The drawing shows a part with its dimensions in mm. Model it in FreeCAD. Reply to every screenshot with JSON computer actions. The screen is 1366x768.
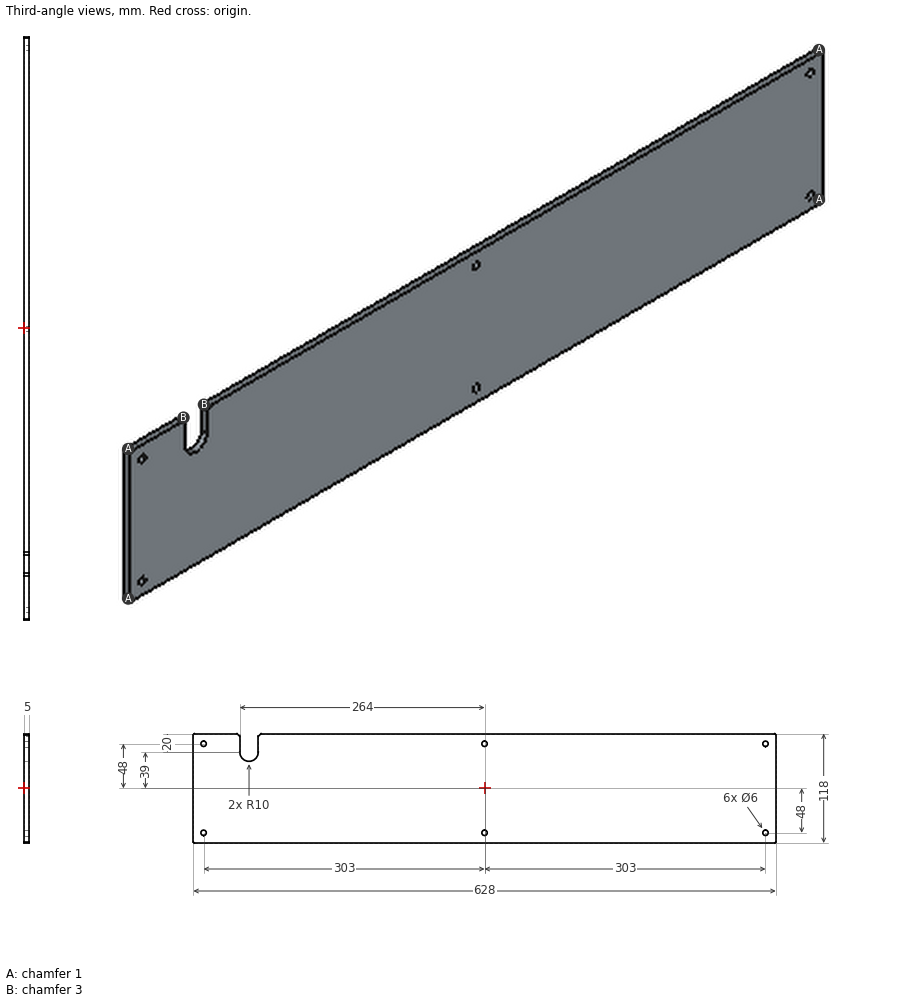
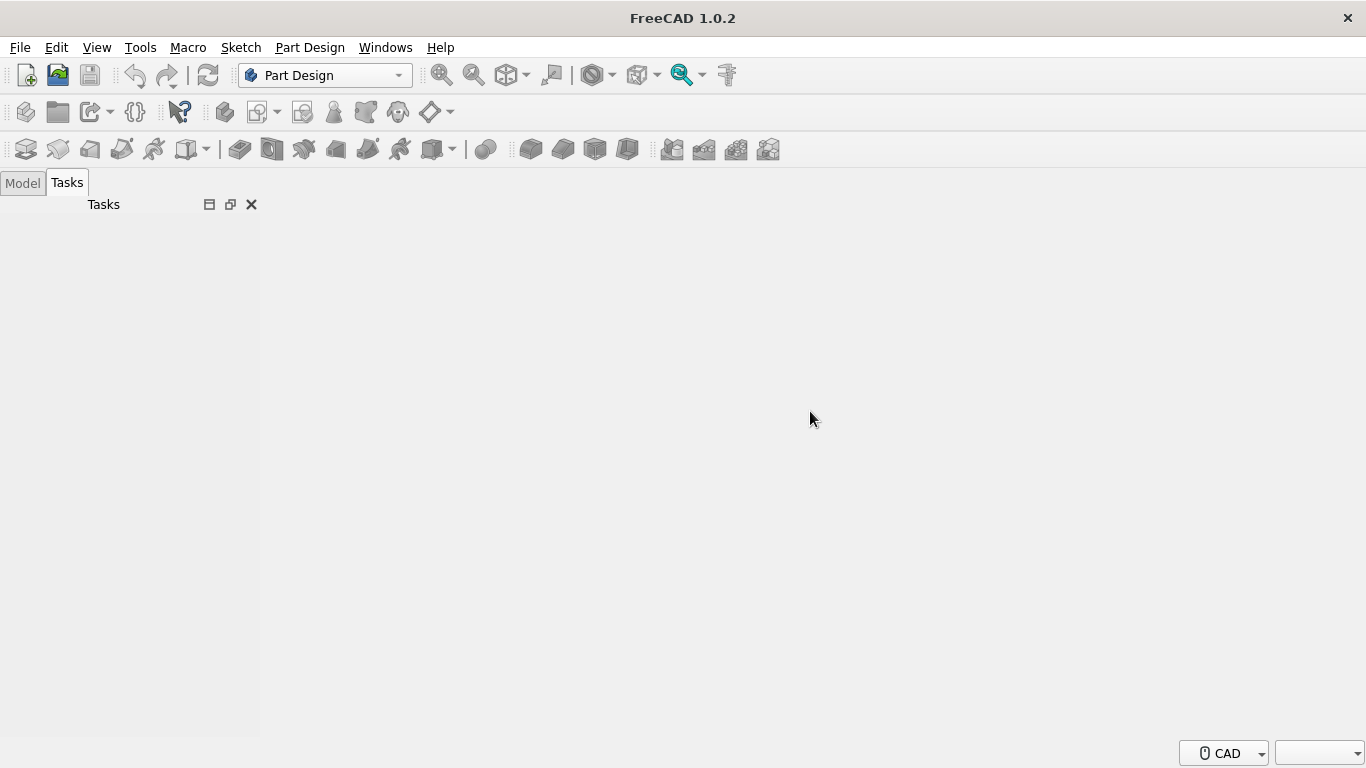
{"action": "key", "text": "ctrl+n"}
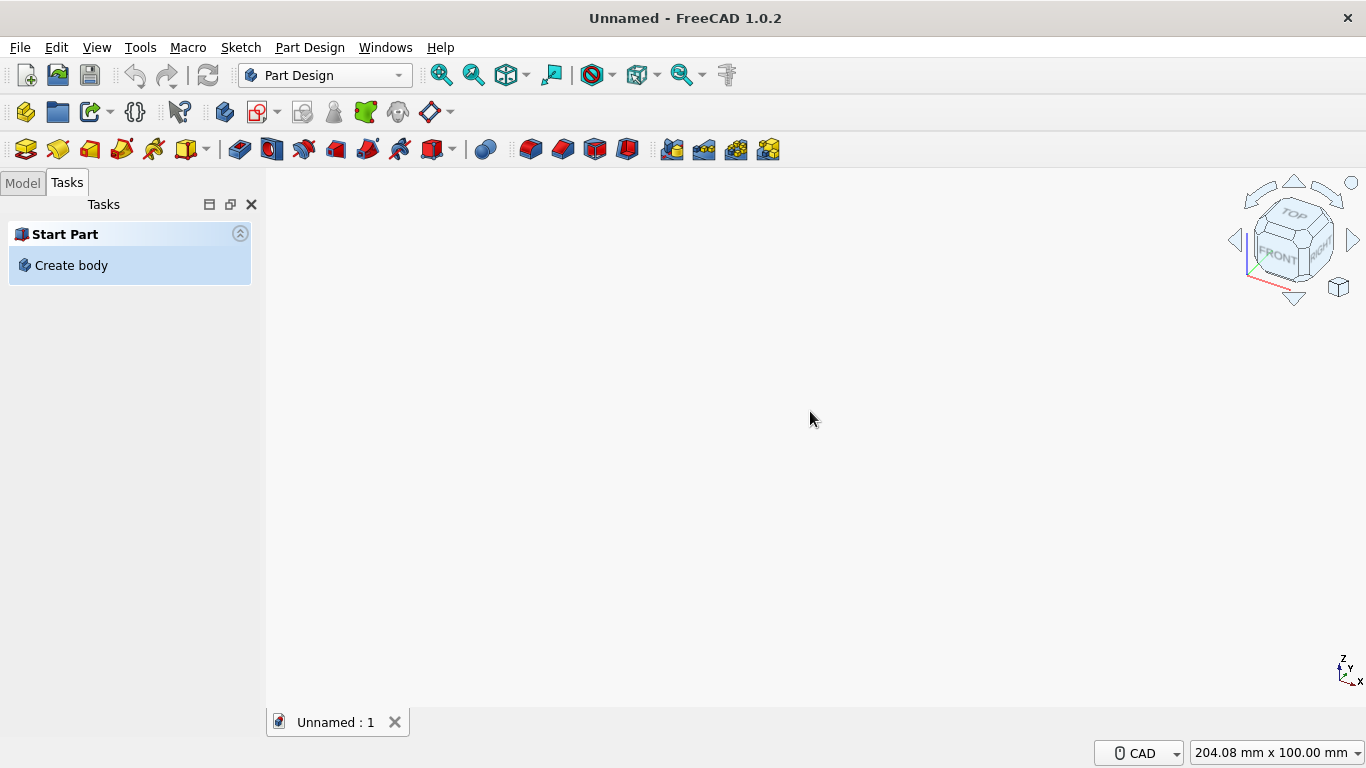
{"action": "left_click", "coordinate": [258, 112]}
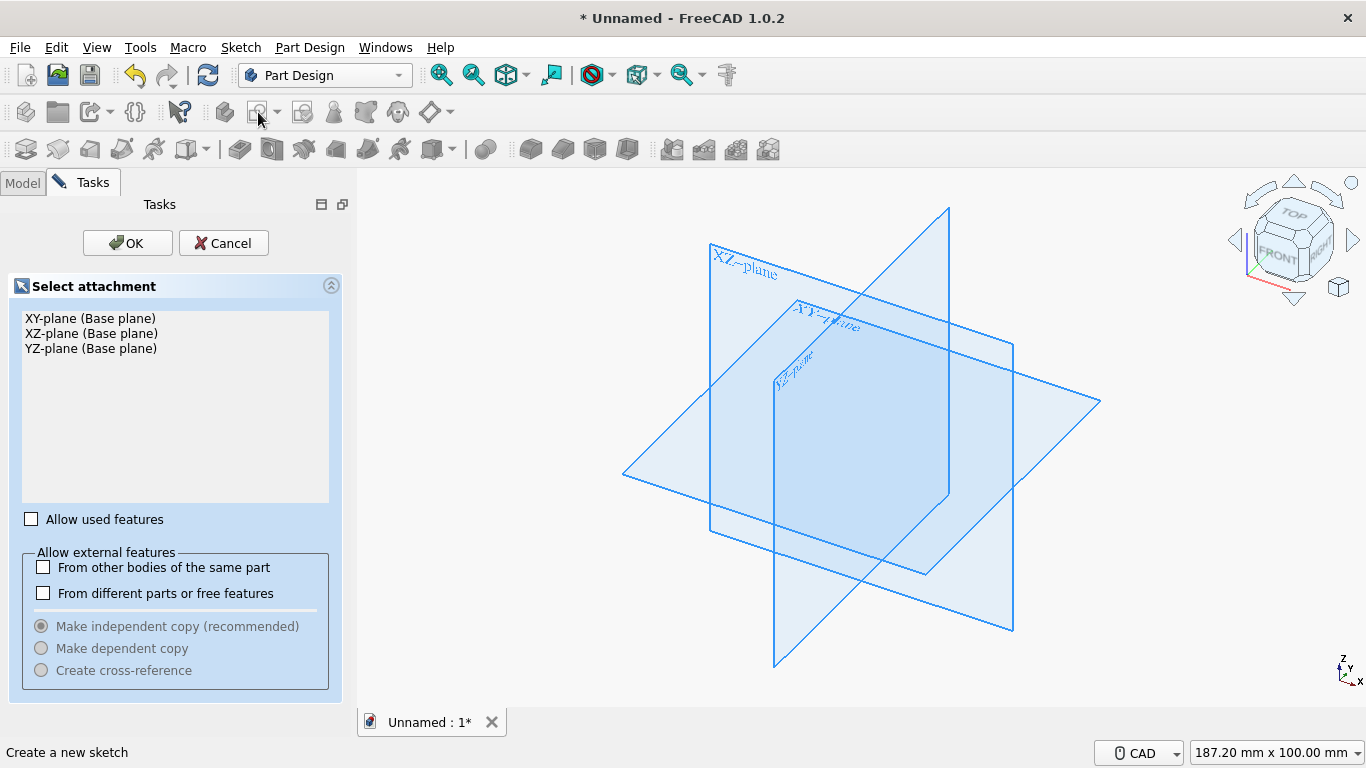
{"action": "left_click", "coordinate": [82, 348]}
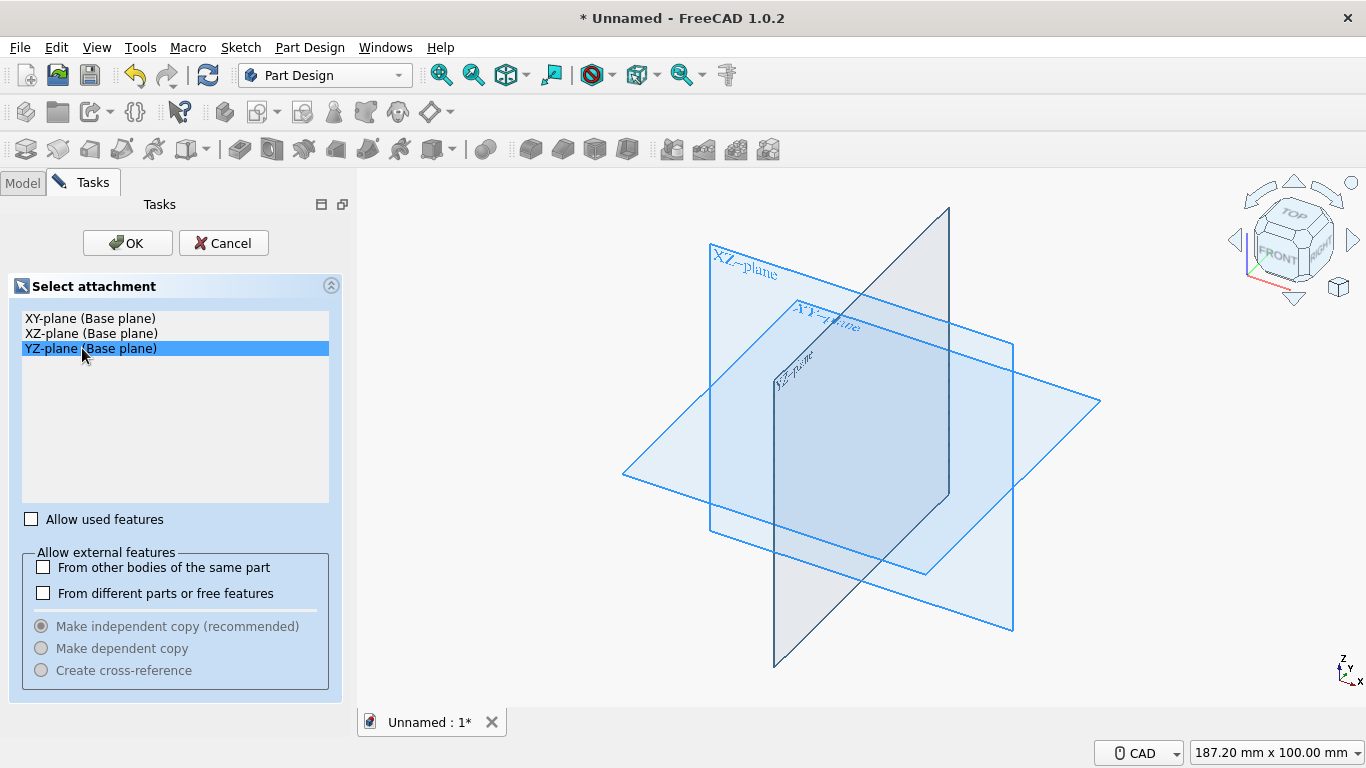
{"action": "left_click", "coordinate": [128, 243]}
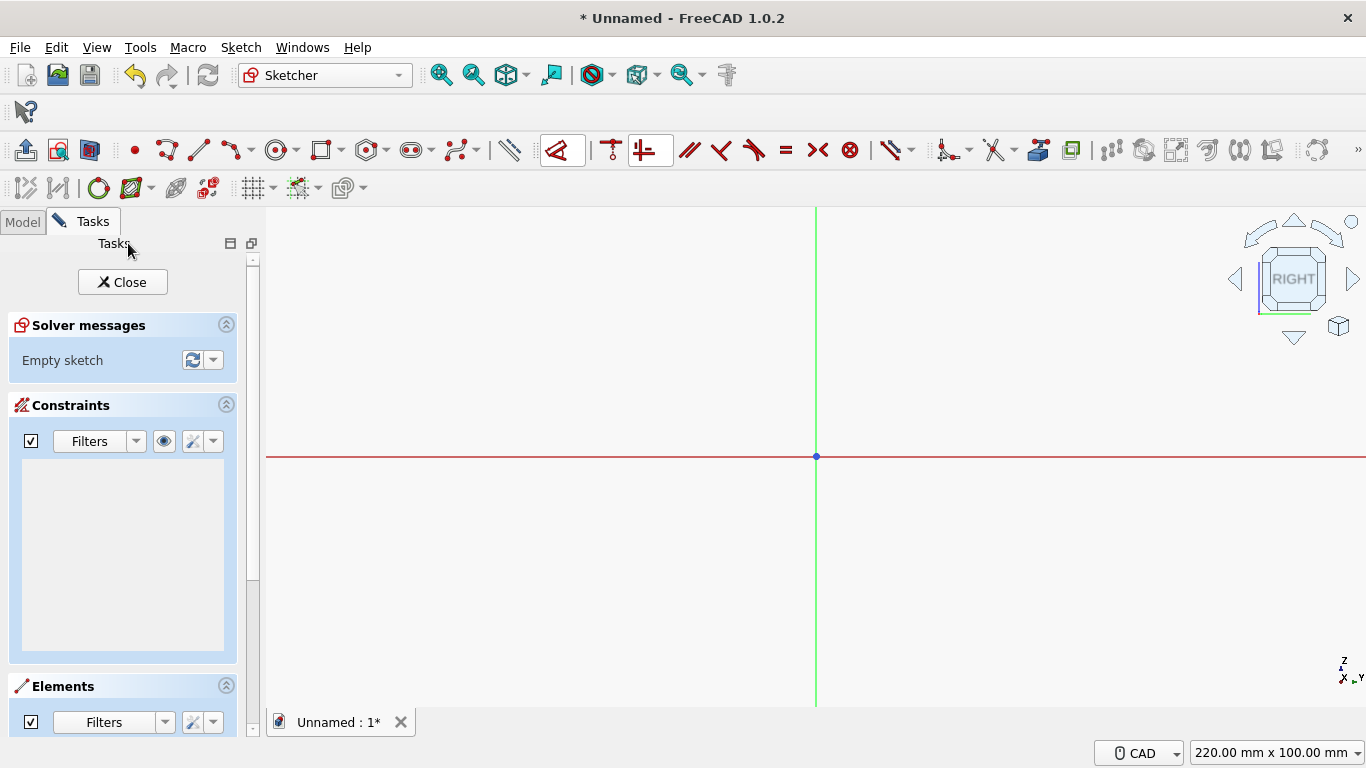
{"action": "scroll", "coordinate": [730, 457], "scroll_direction": "down", "scroll_amount": 8}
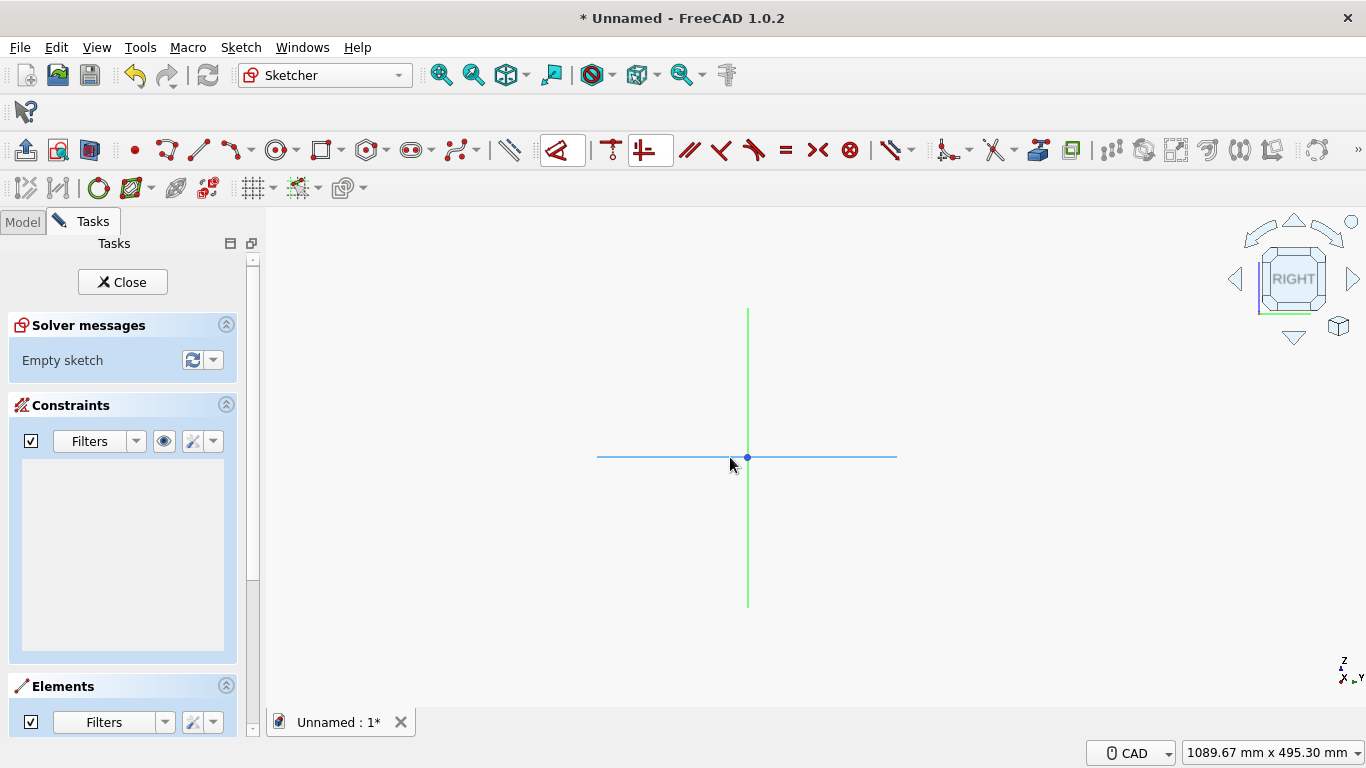
{"action": "key", "text": "g v"}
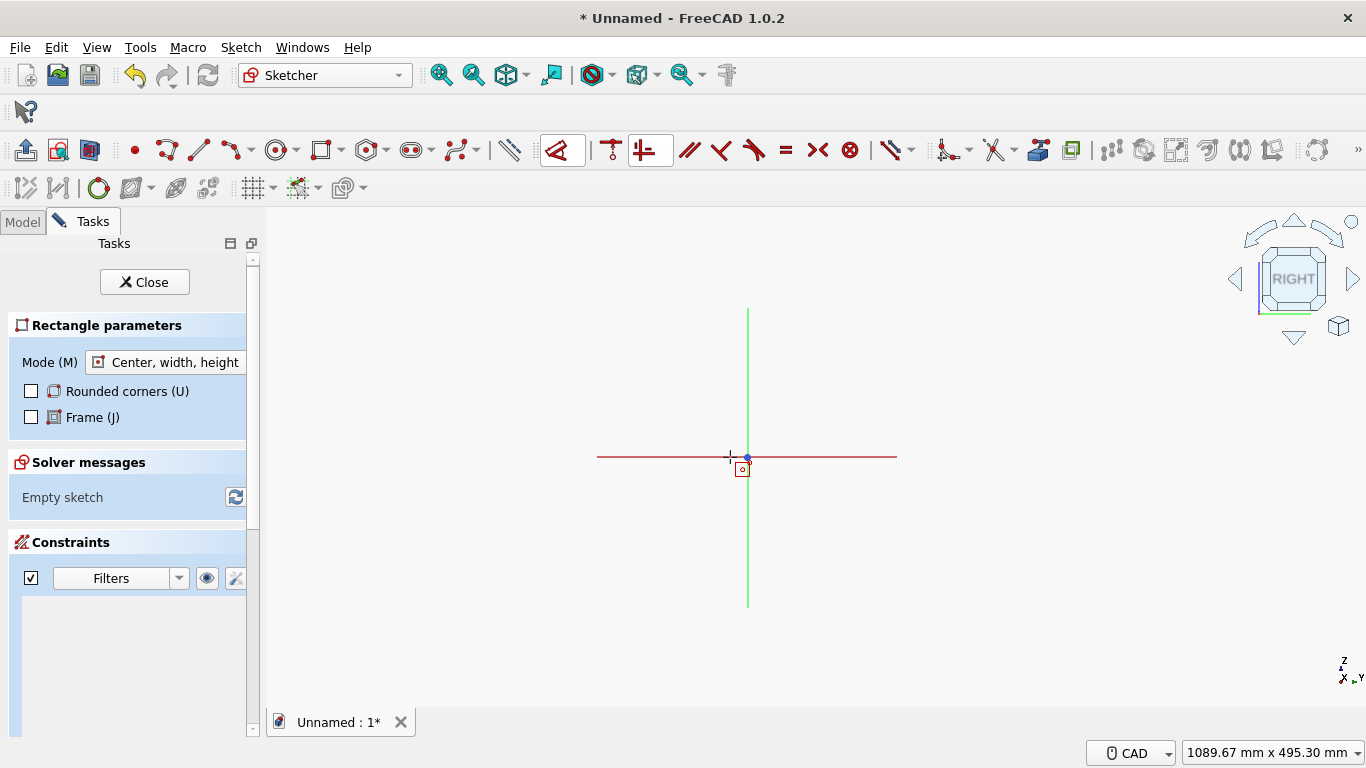
{"action": "left_click", "coordinate": [748, 457]}
{"action": "mouse_move", "coordinate": [1065, 398]}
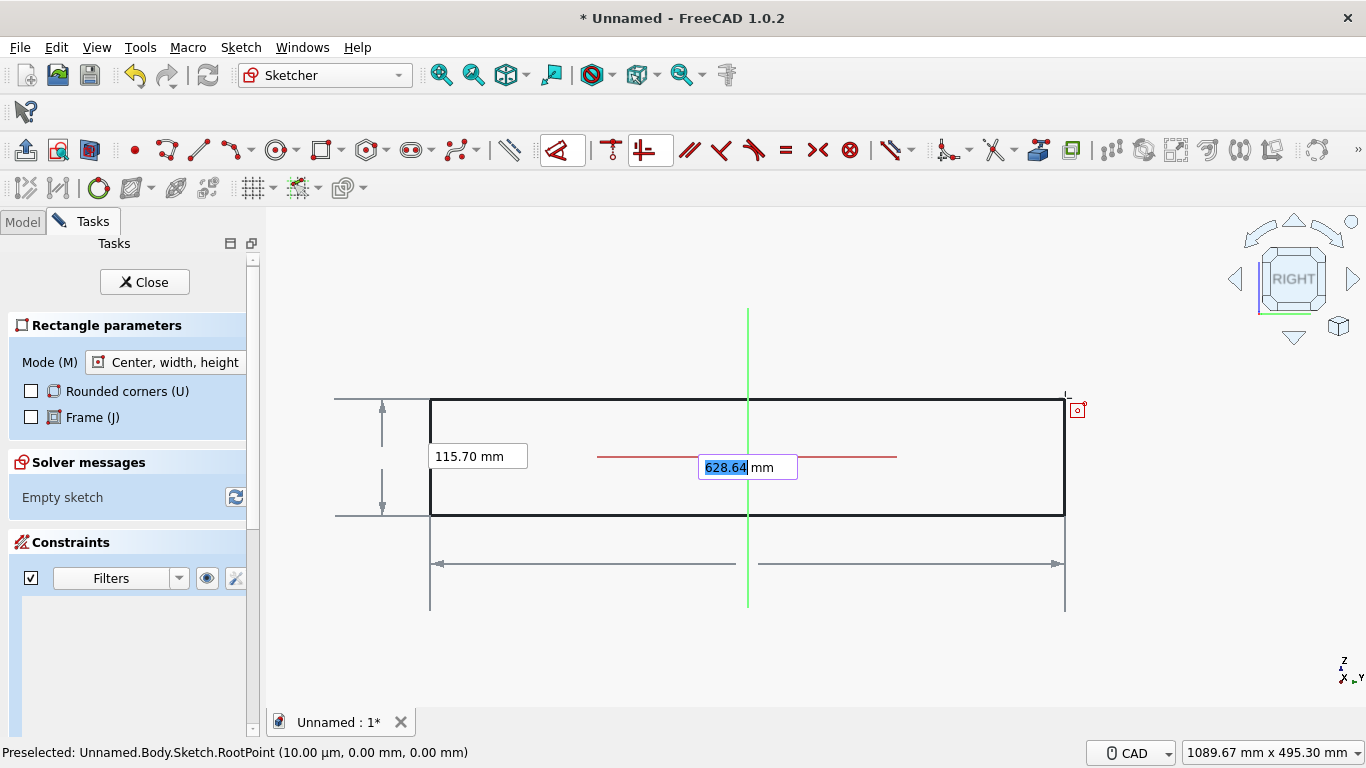
{"action": "type", "text": "628"}
{"action": "key", "text": "Tab"}
{"action": "type", "text": "118"}
{"action": "key", "text": "Return"}
{"action": "key", "text": "Escape"}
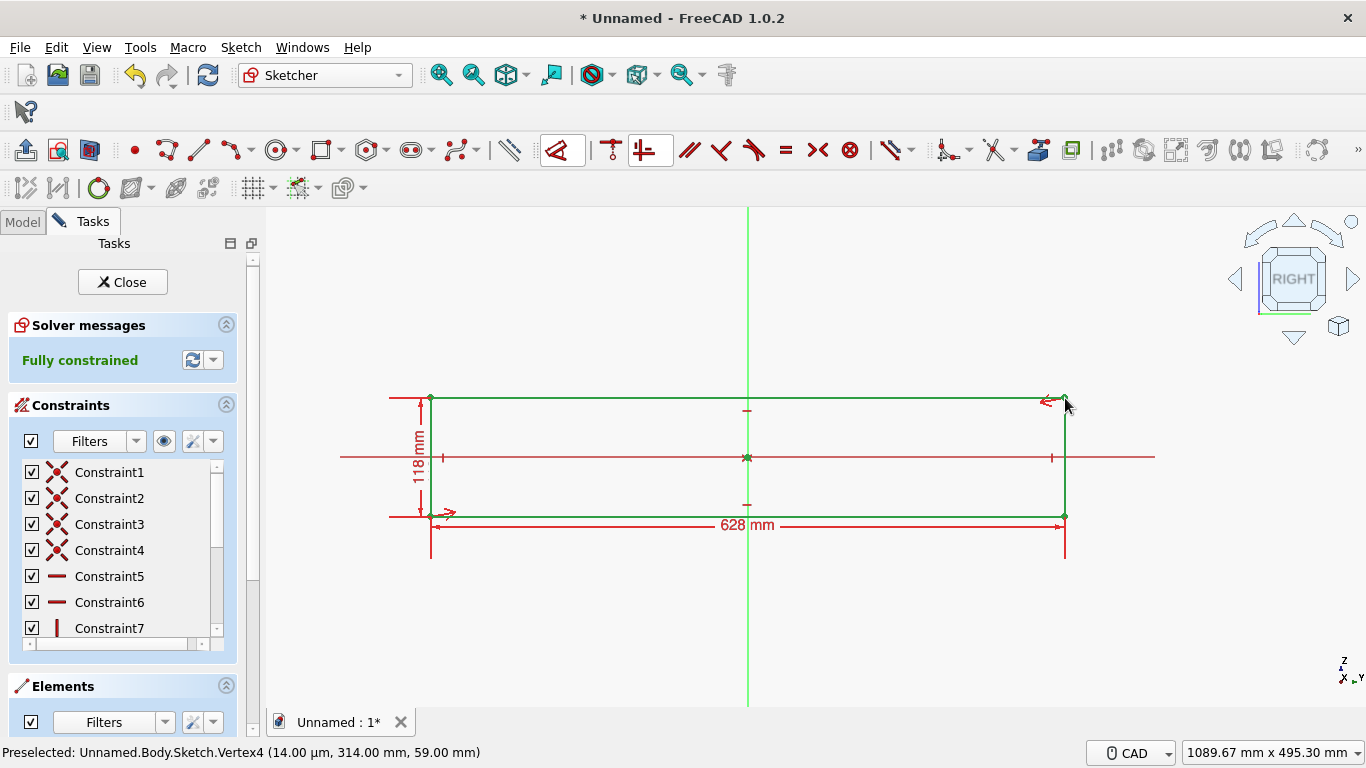
{"action": "left_click", "coordinate": [123, 282]}